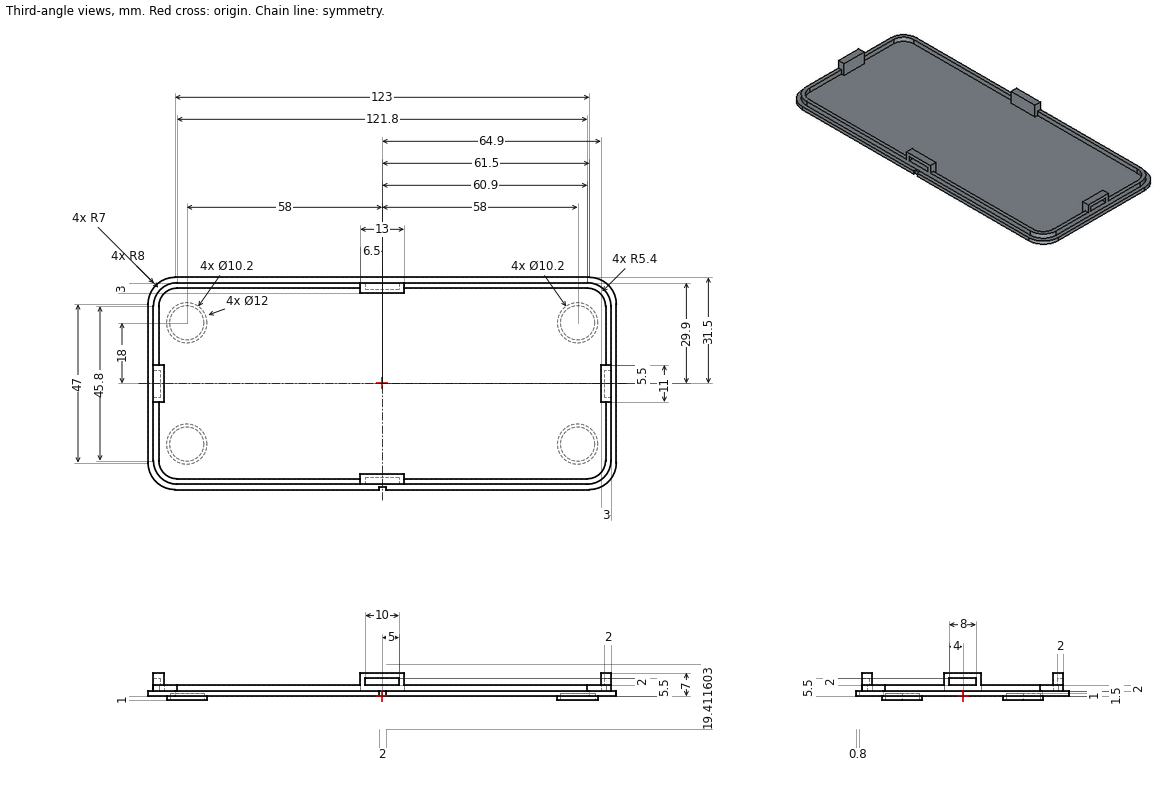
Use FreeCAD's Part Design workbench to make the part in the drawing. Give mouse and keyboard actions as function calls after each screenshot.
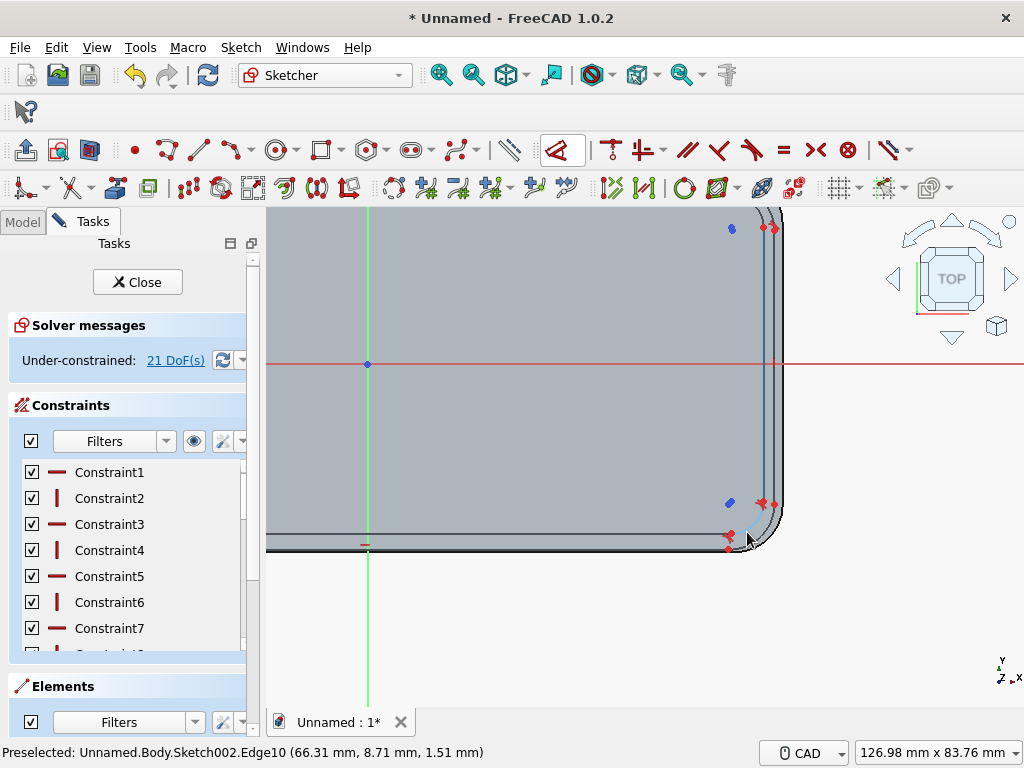
click(746, 530)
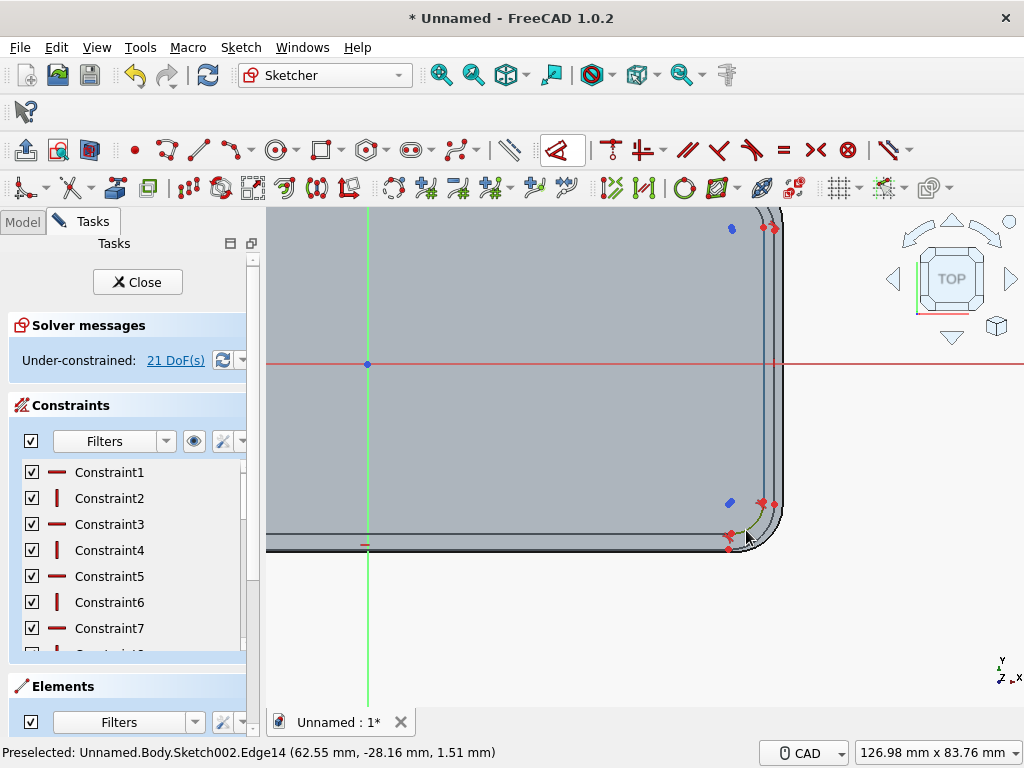
key(t)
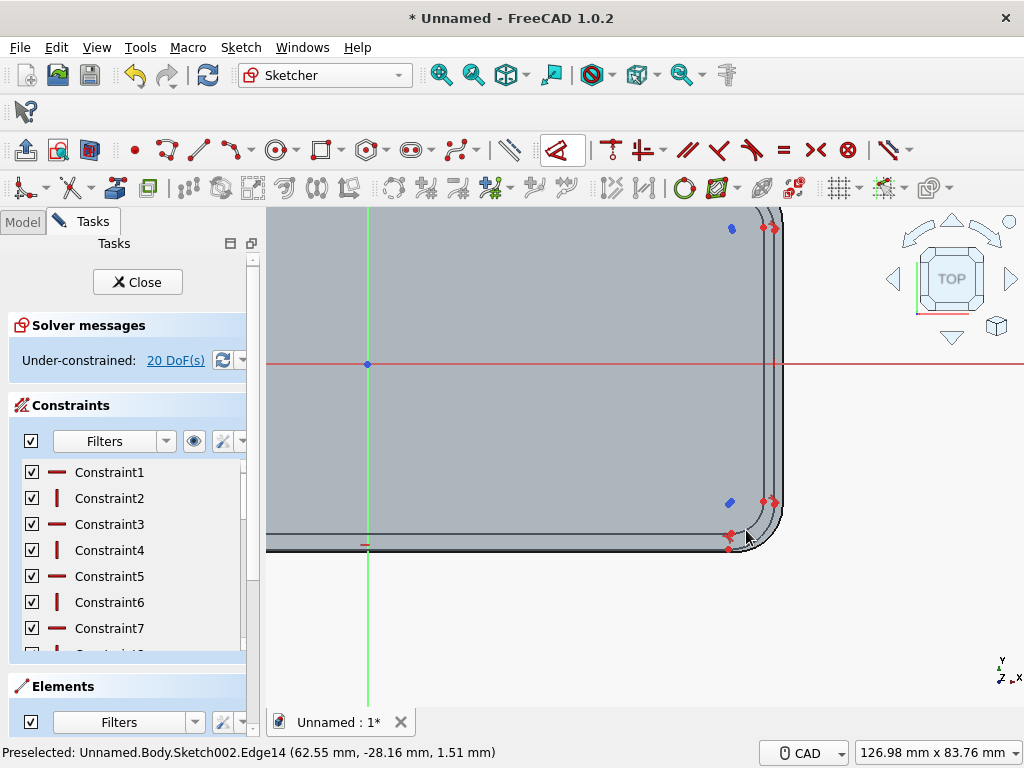
click(513, 534)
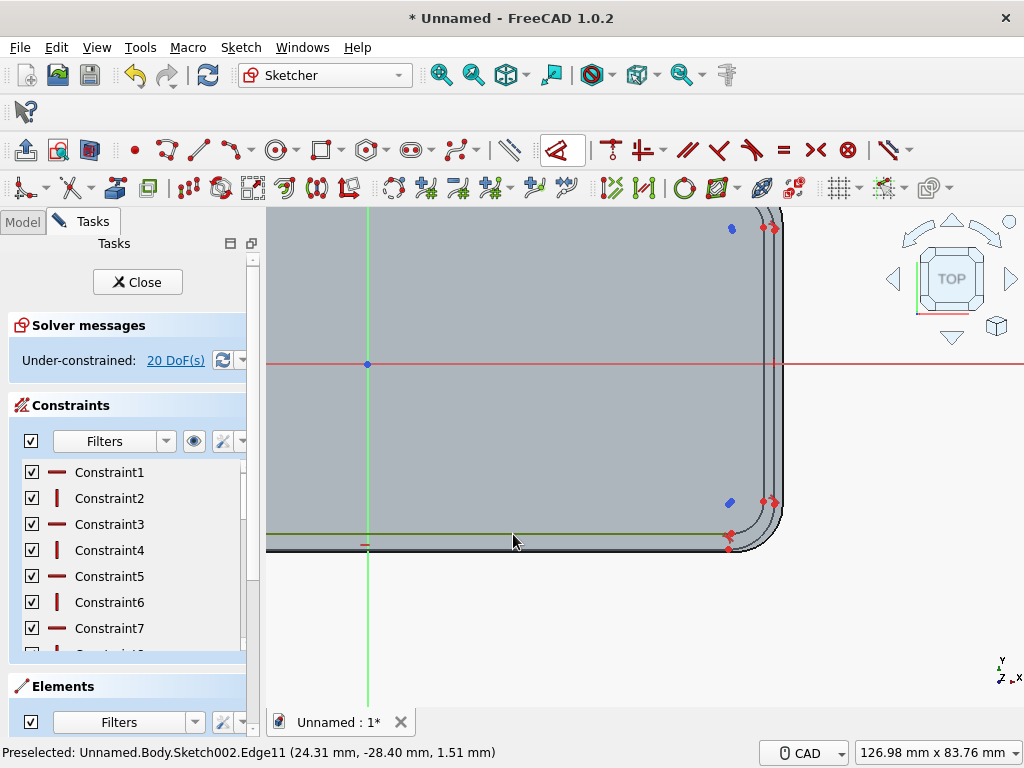
click(746, 530)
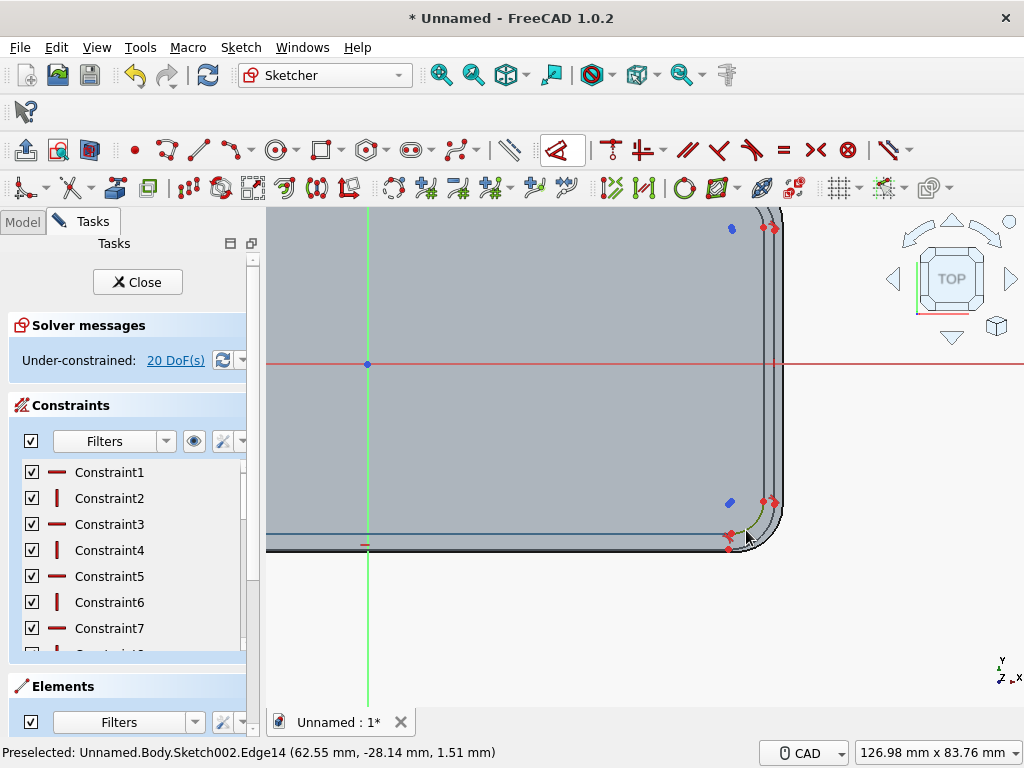
key(t)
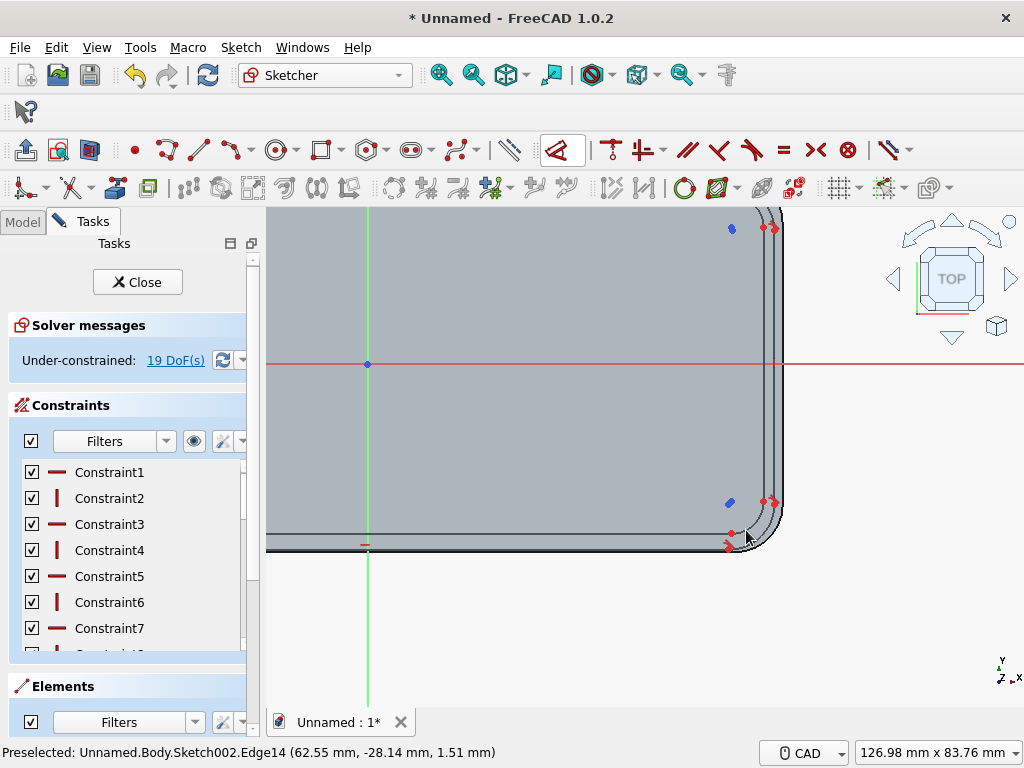
click(513, 534)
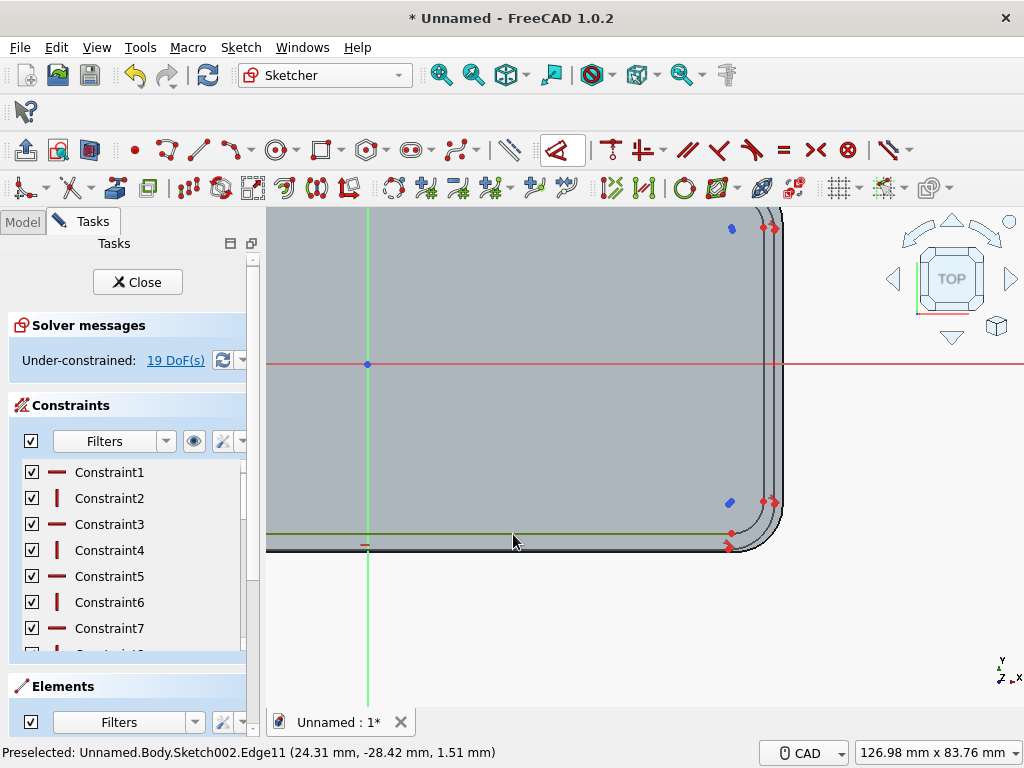
scroll(747, 533, down, 4)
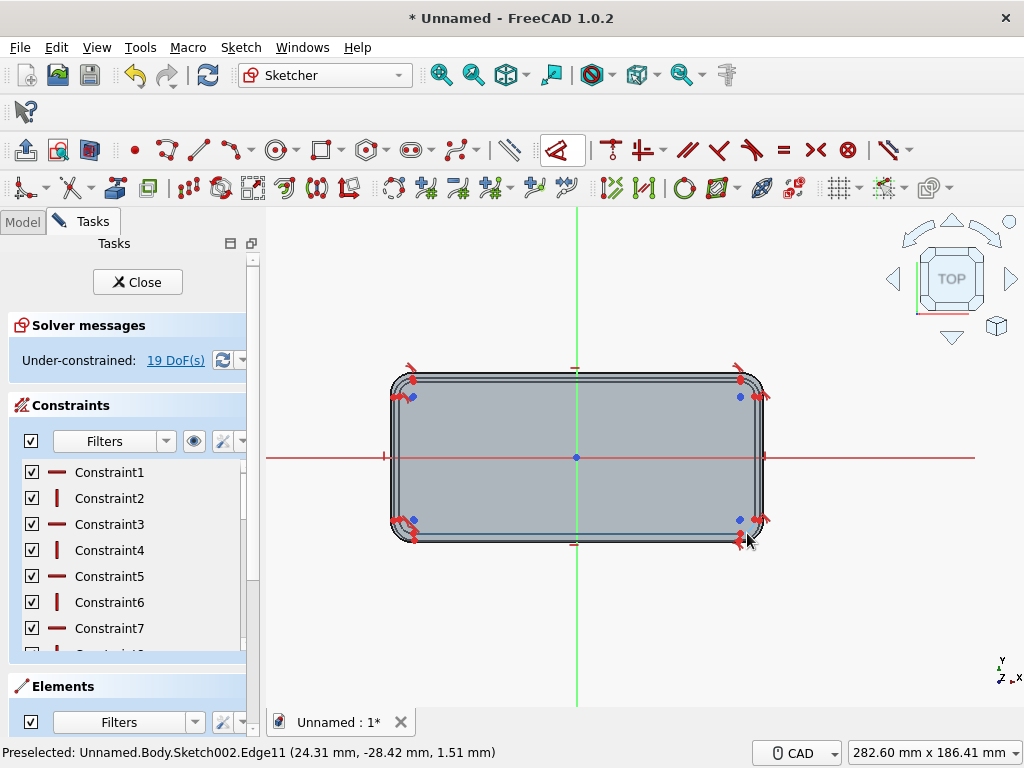
scroll(401, 526, up, 5)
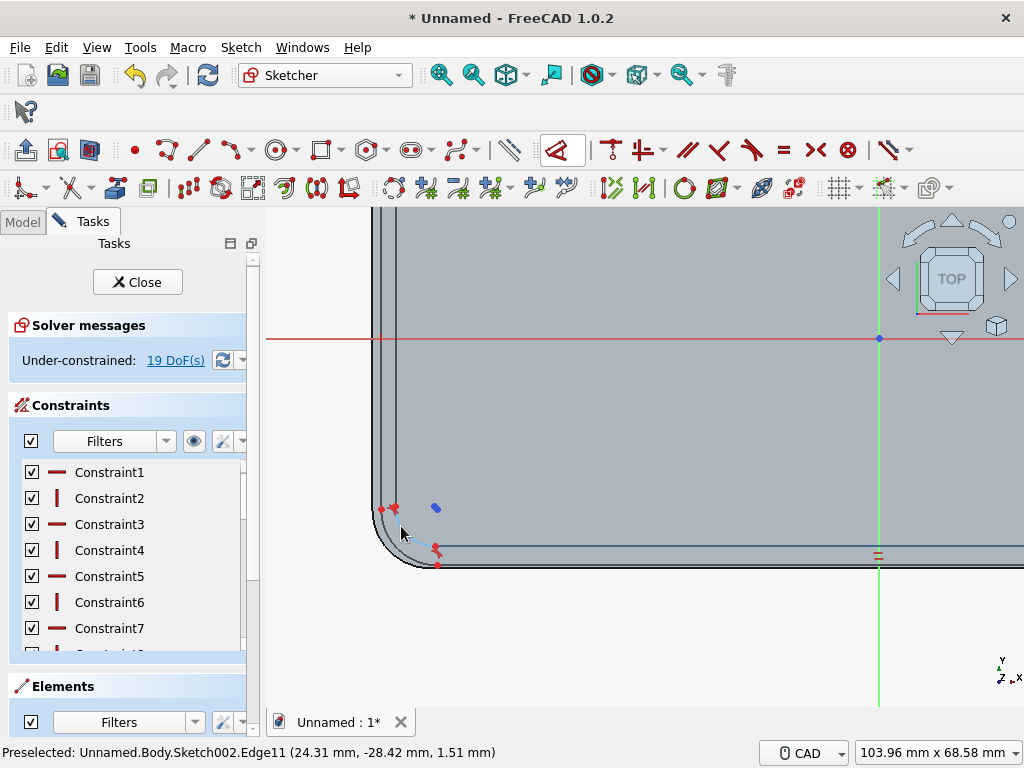
click(400, 524)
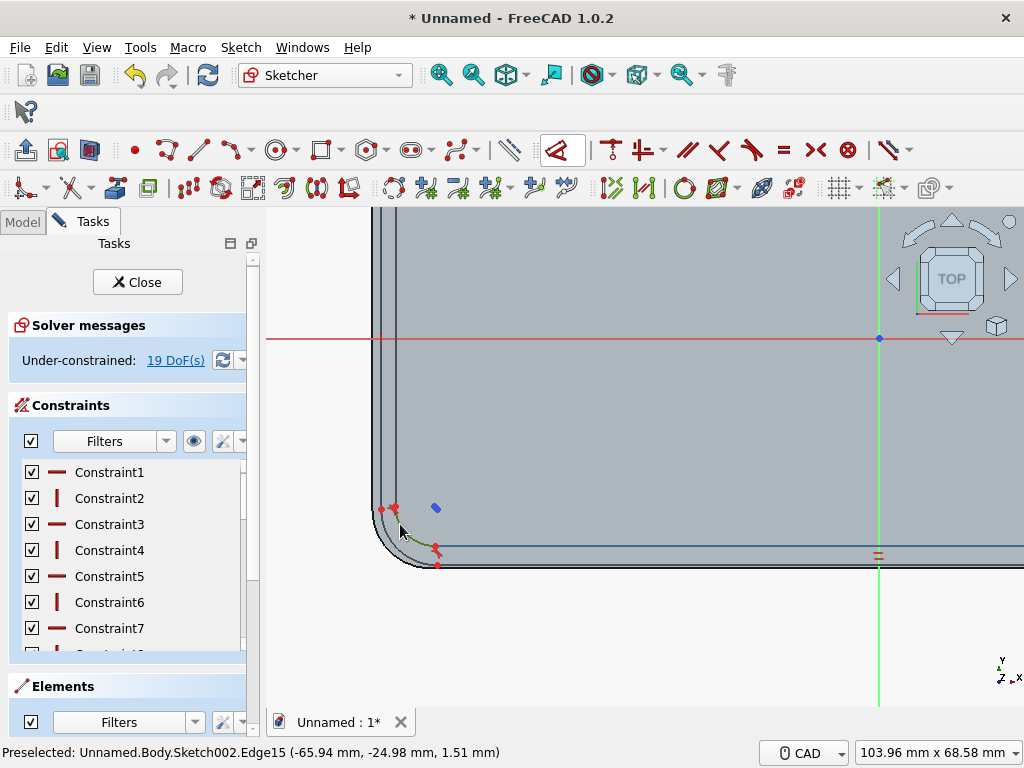
key(t)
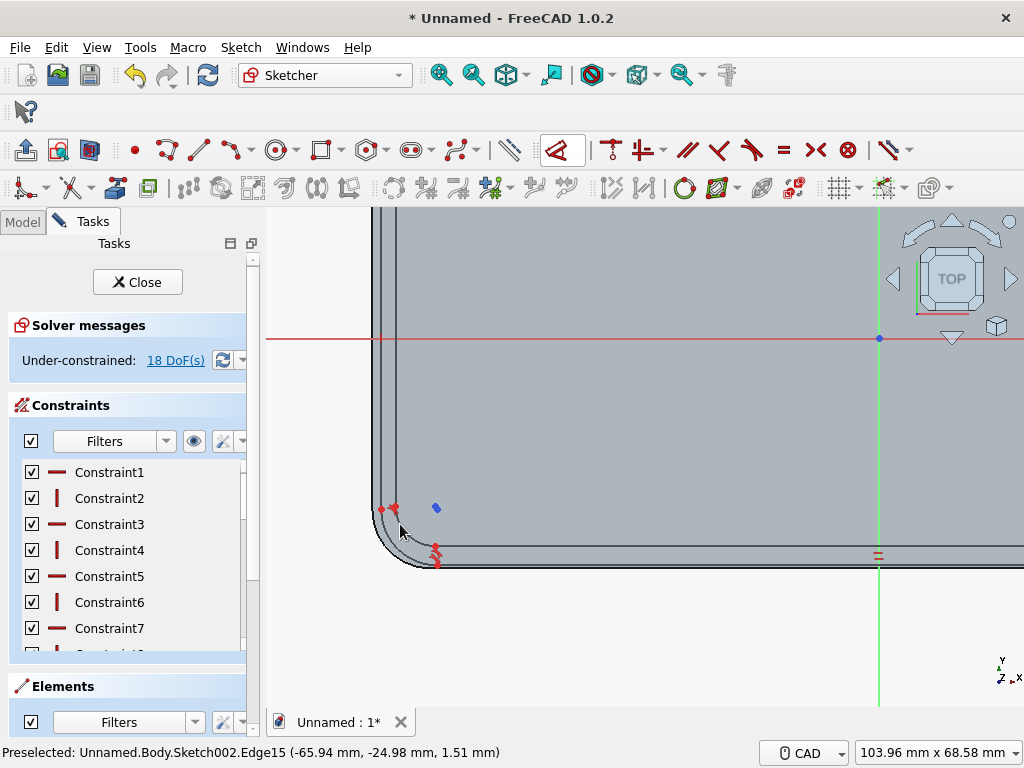
click(396, 406)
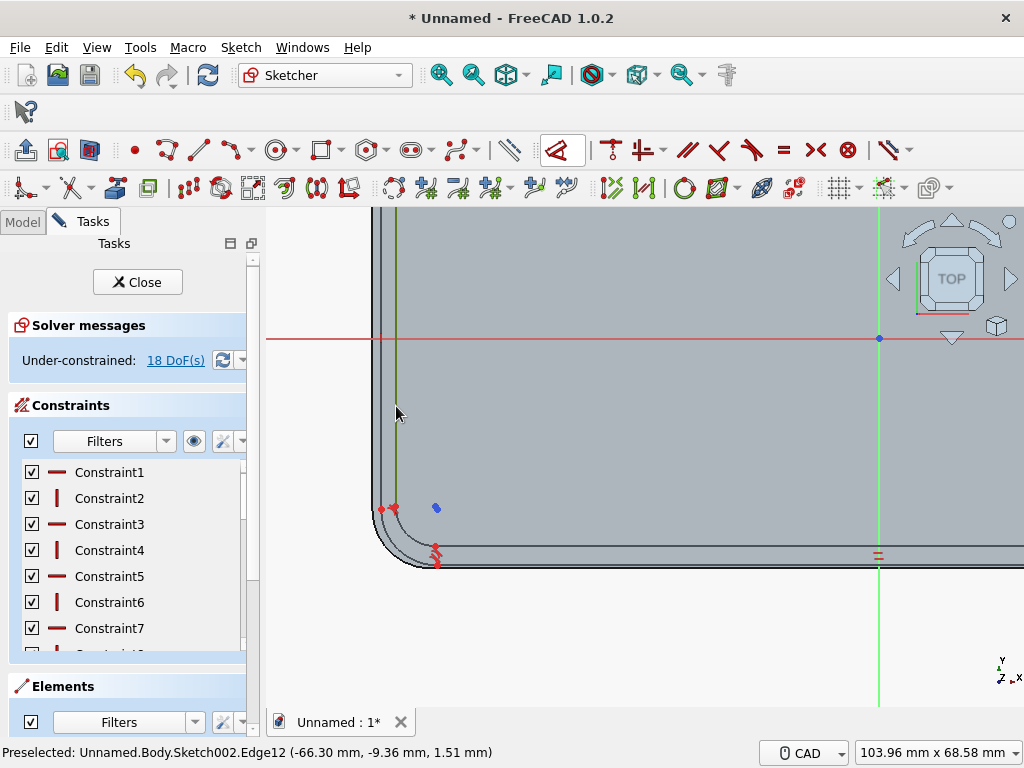
click(400, 524)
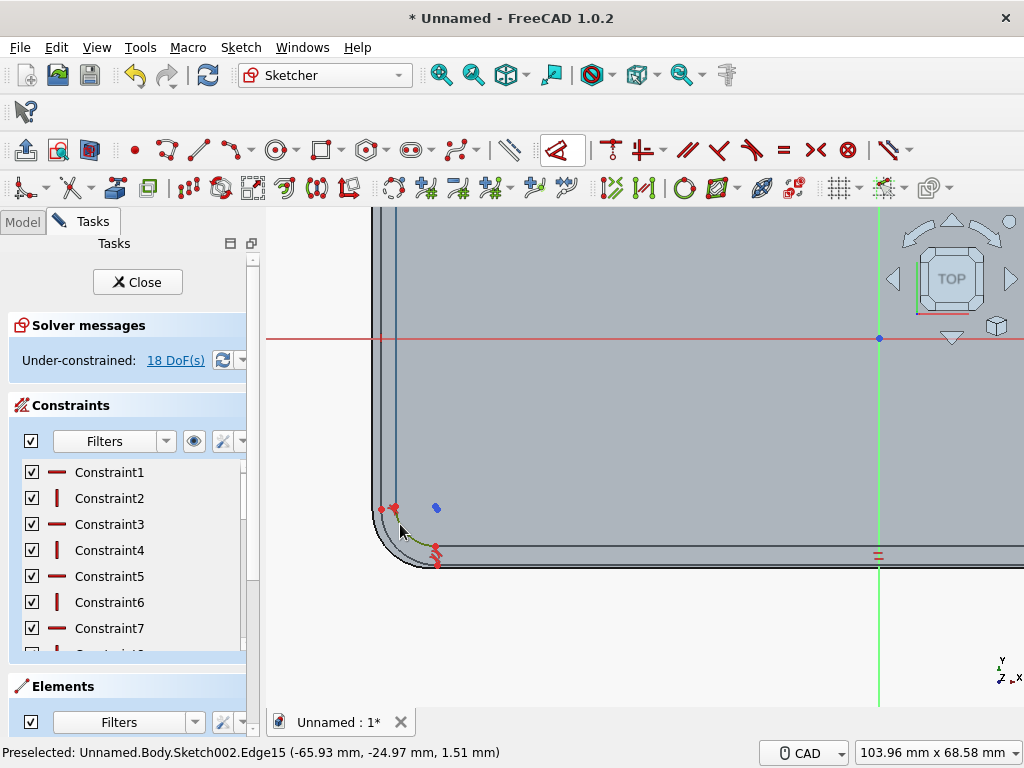
click(752, 150)